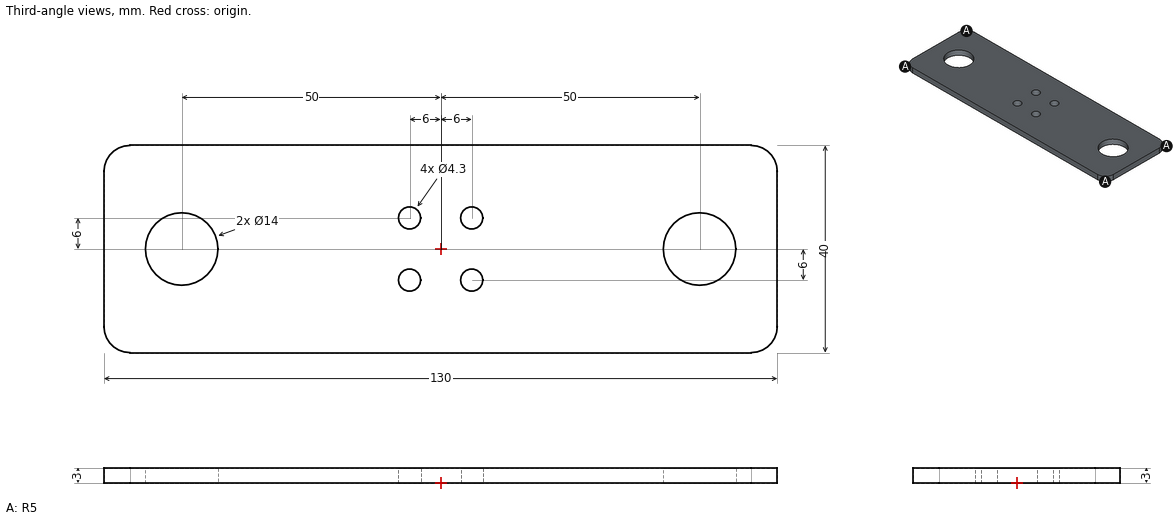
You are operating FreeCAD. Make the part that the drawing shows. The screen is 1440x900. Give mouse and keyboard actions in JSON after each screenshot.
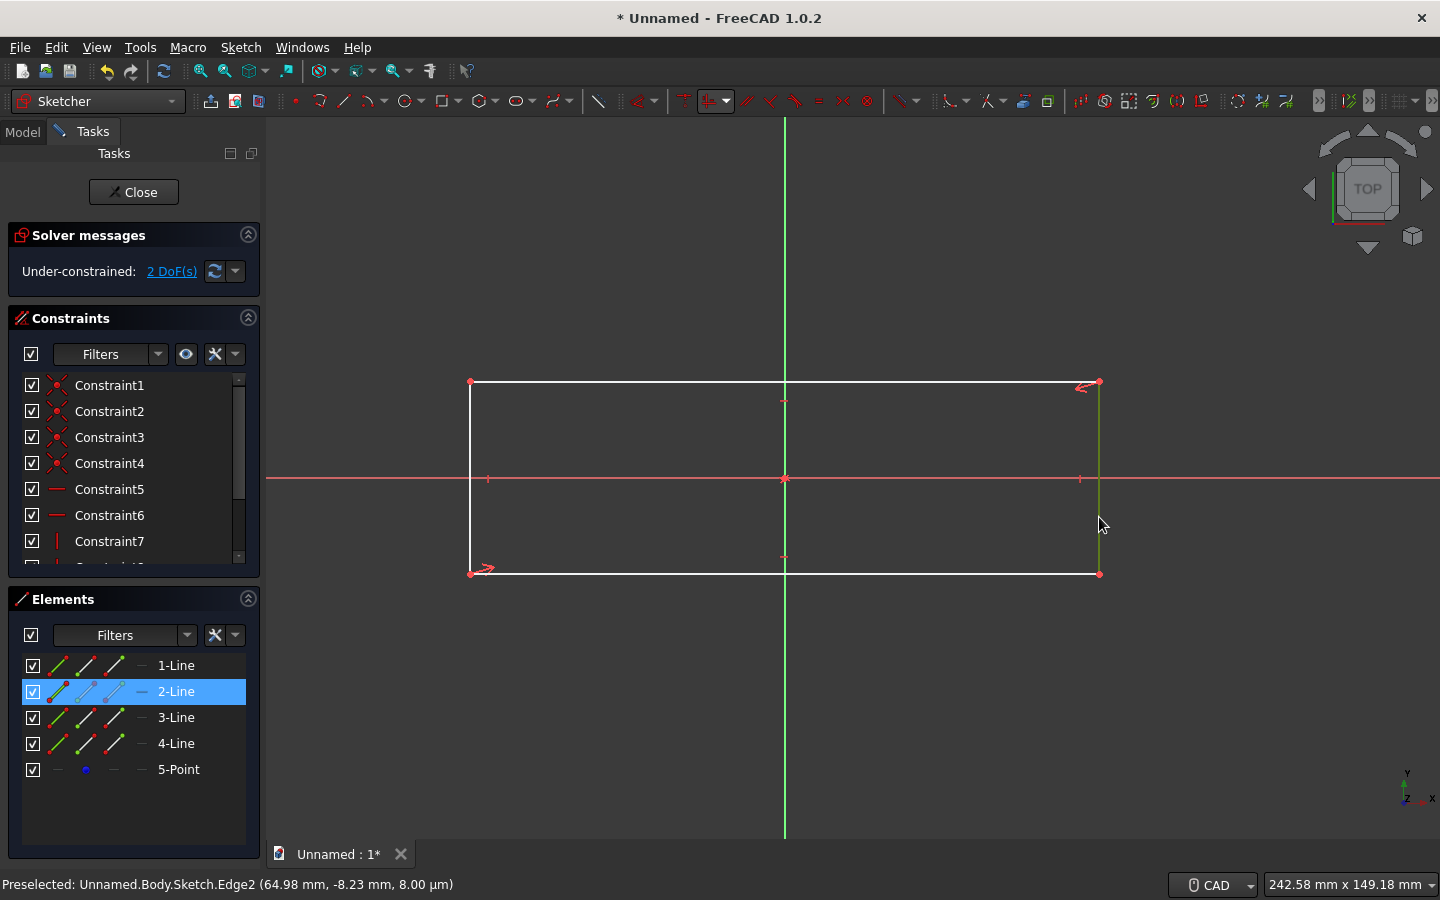
{"action": "key", "text": "i"}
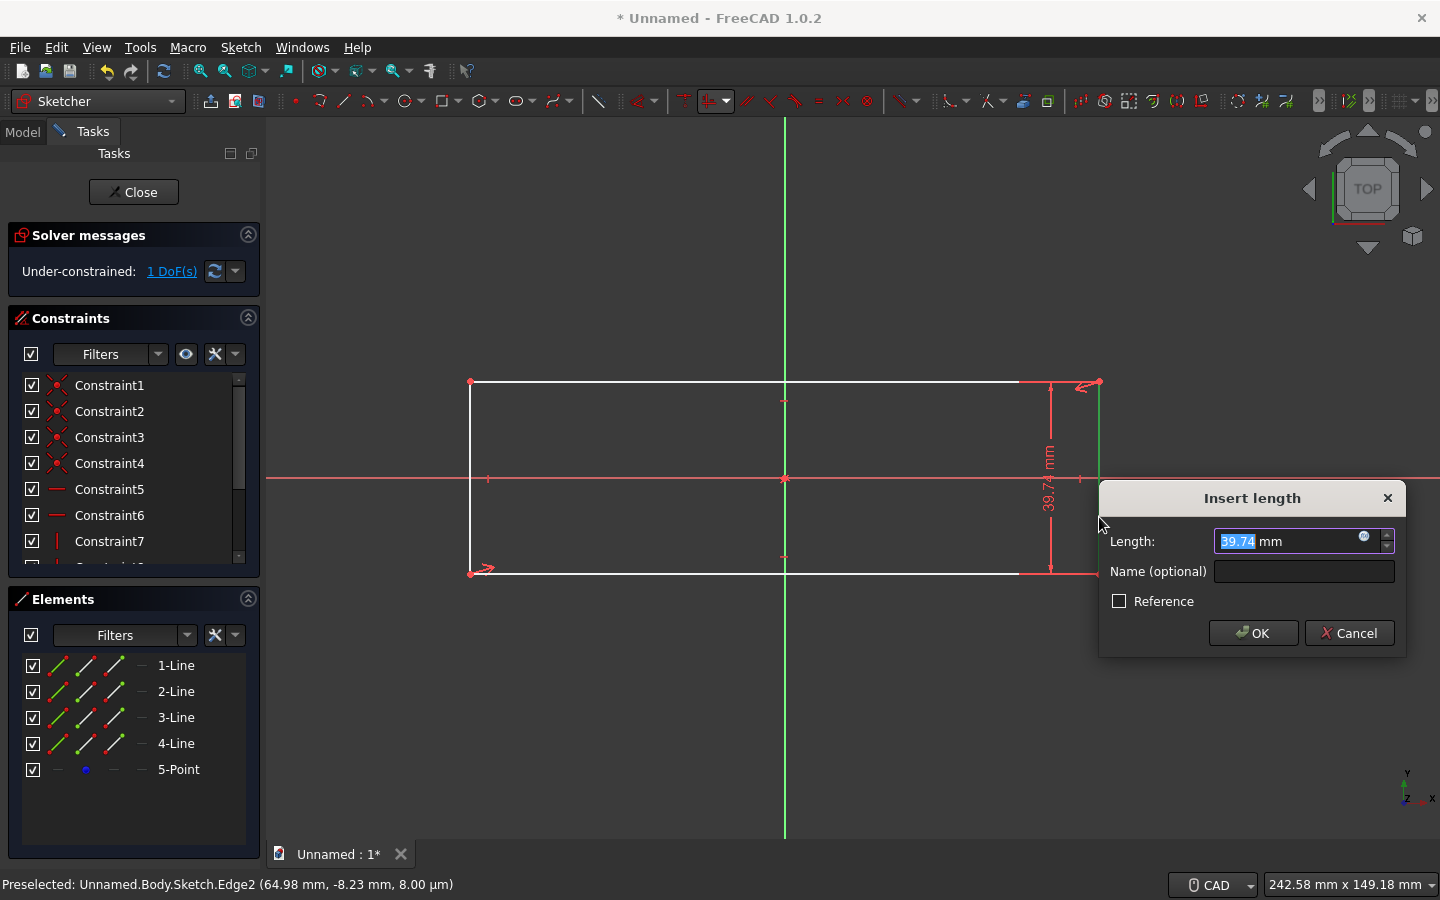
{"action": "type", "text": "40"}
{"action": "key", "text": "Return"}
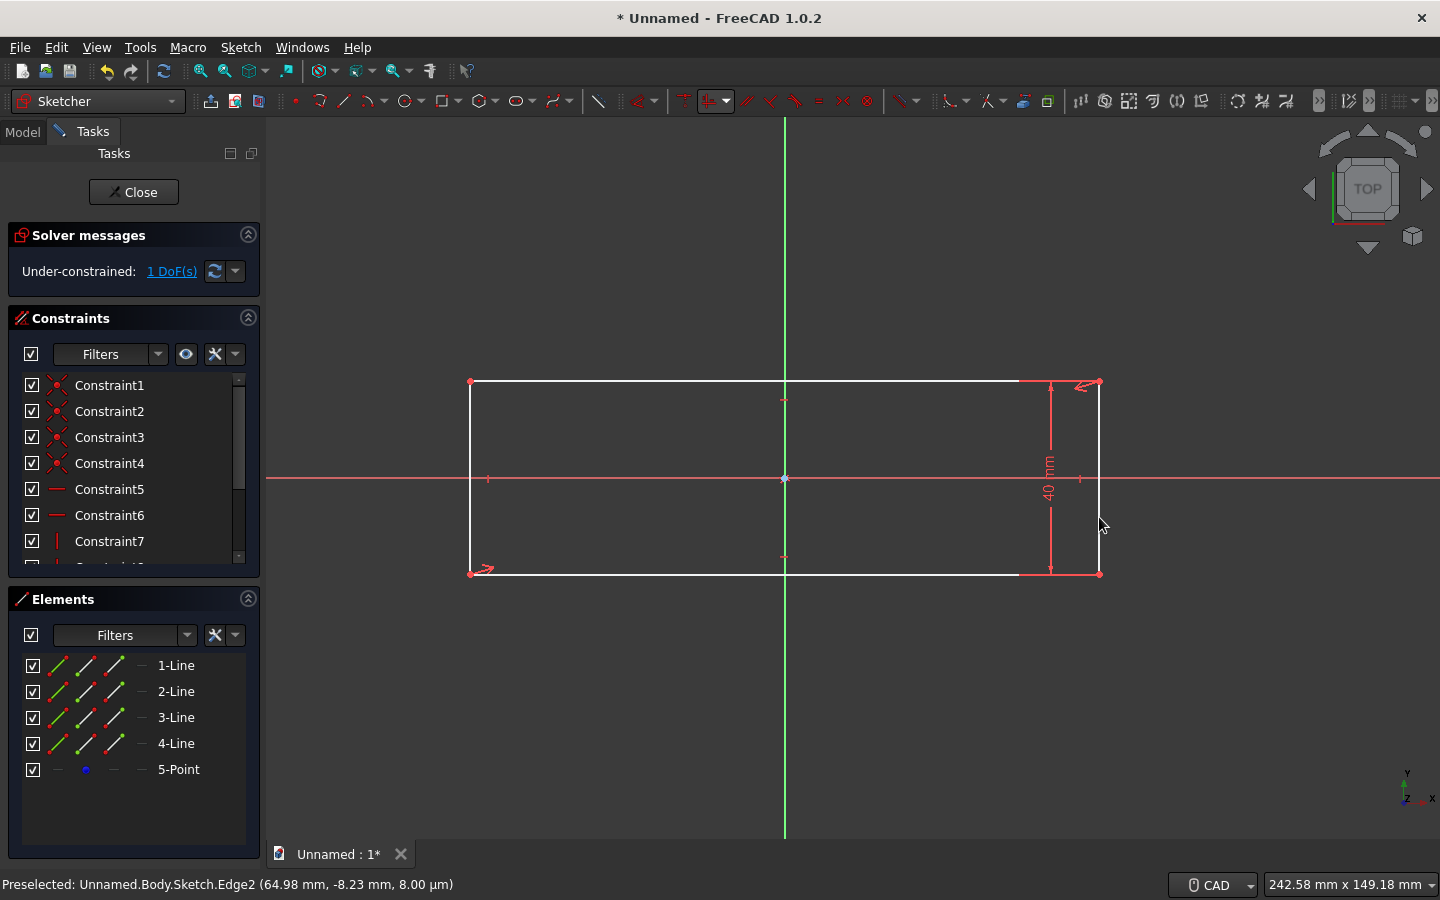
{"action": "left_click", "coordinate": [659, 575]}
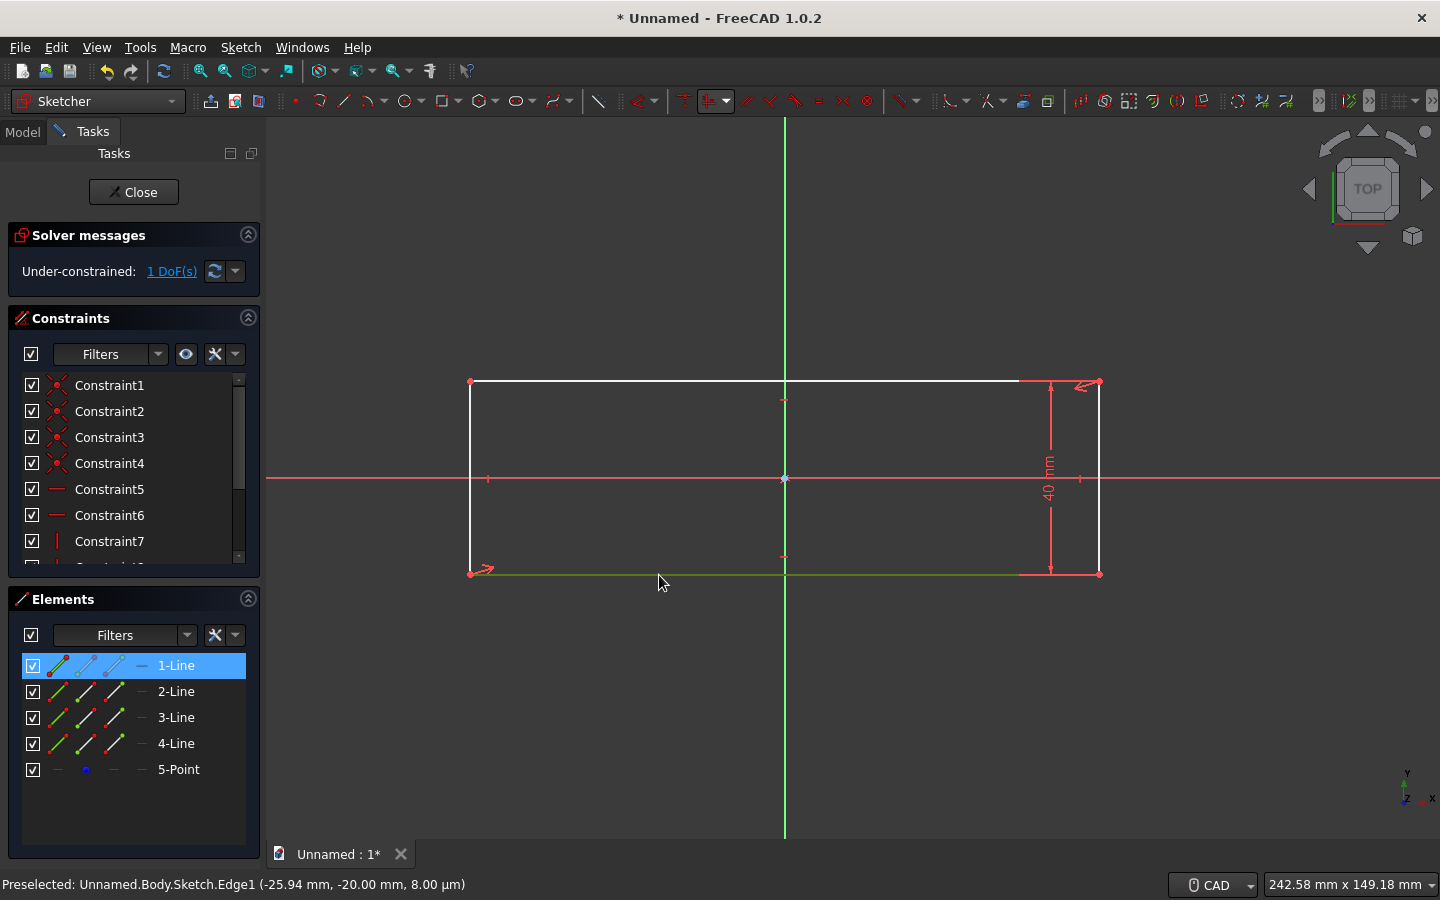
{"action": "key", "text": "l"}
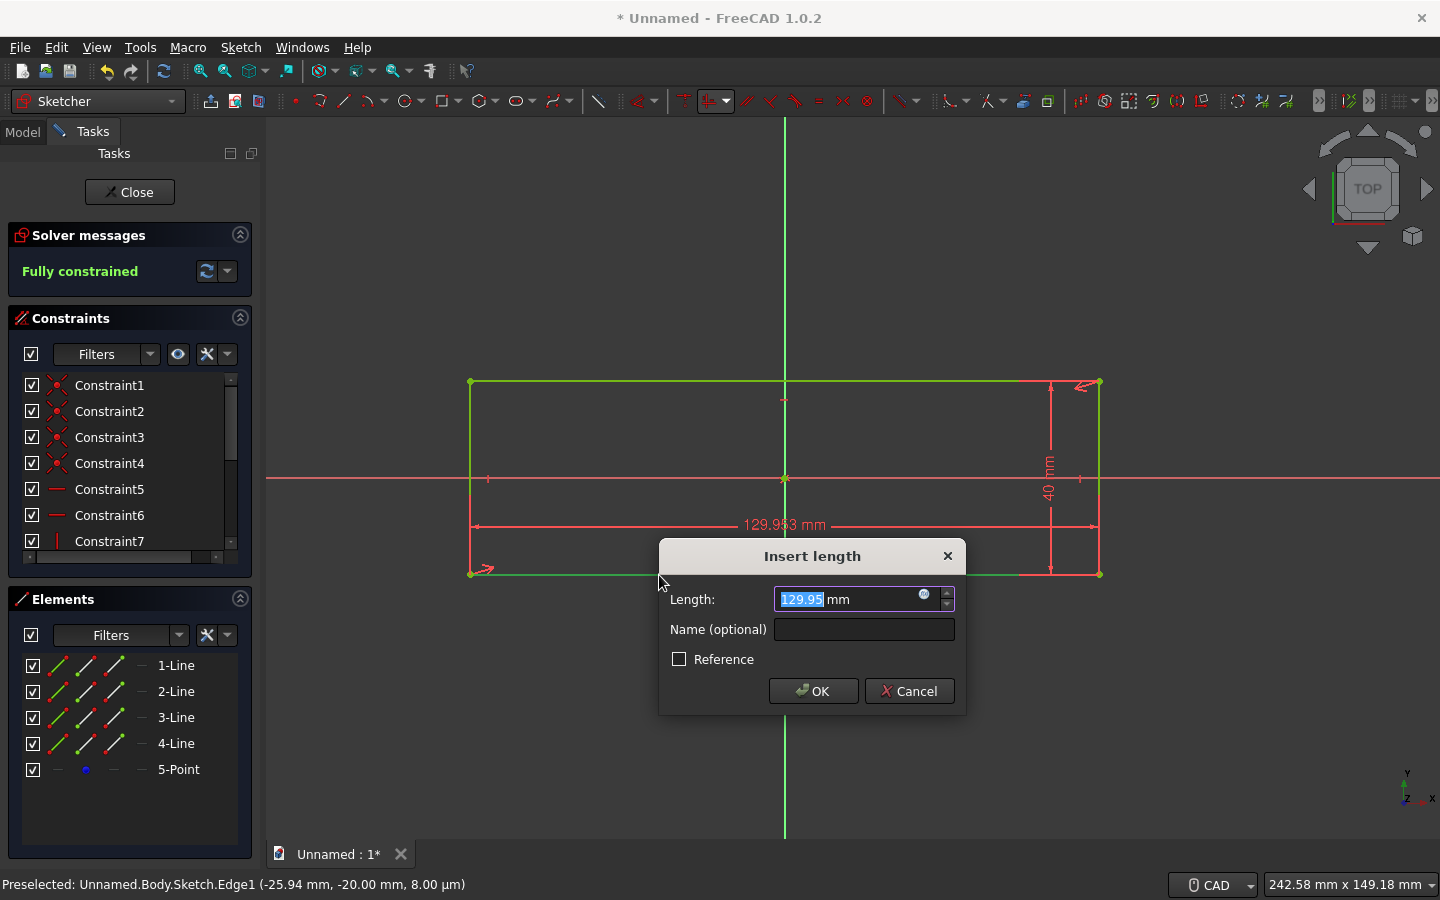
{"action": "type", "text": "130"}
{"action": "key", "text": "Return"}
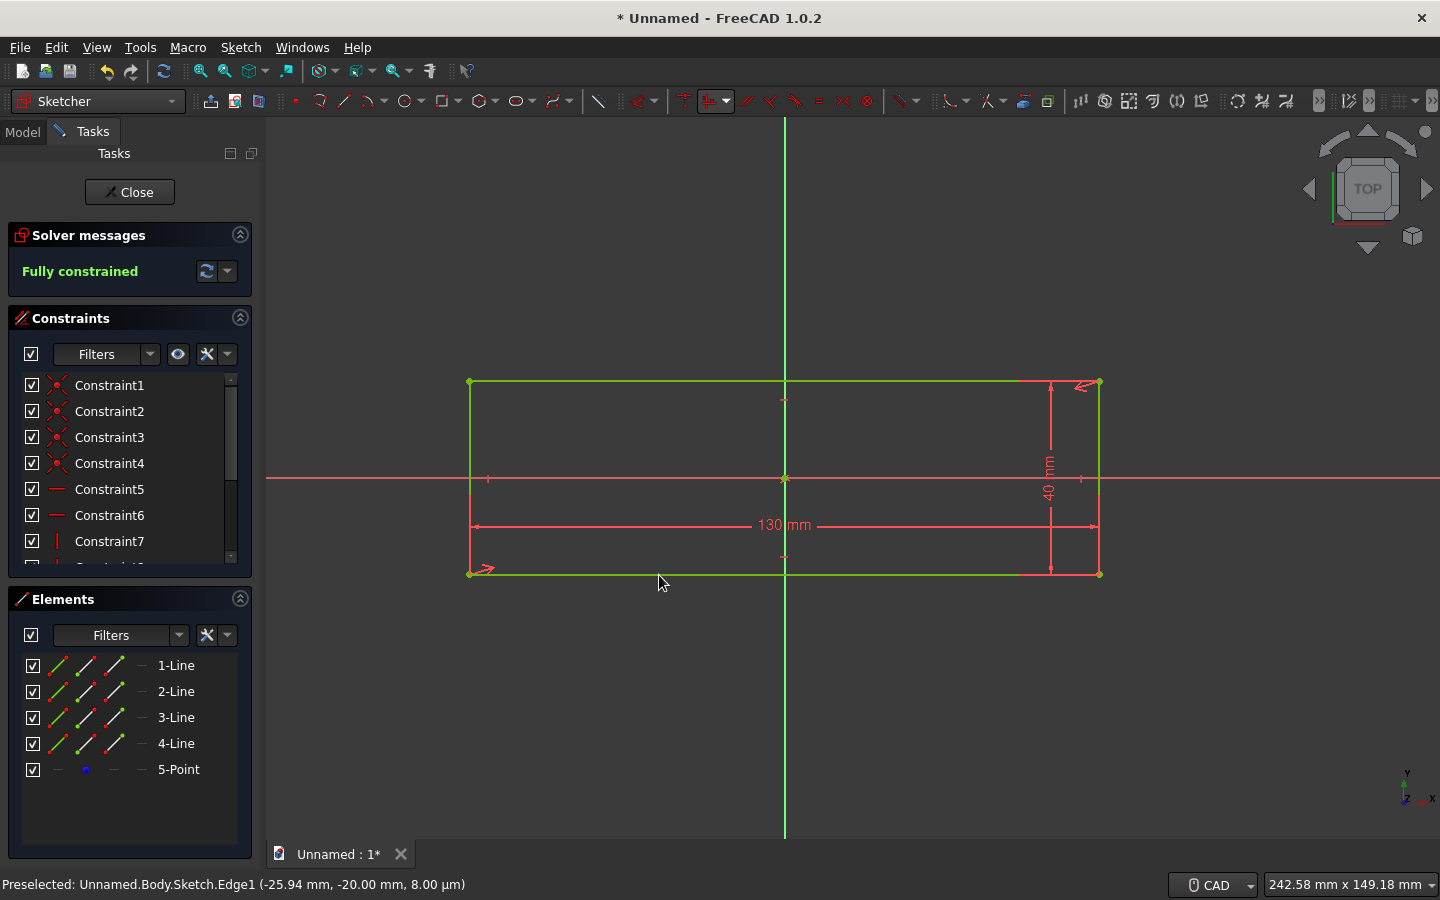
{"action": "left_click", "coordinate": [130, 192]}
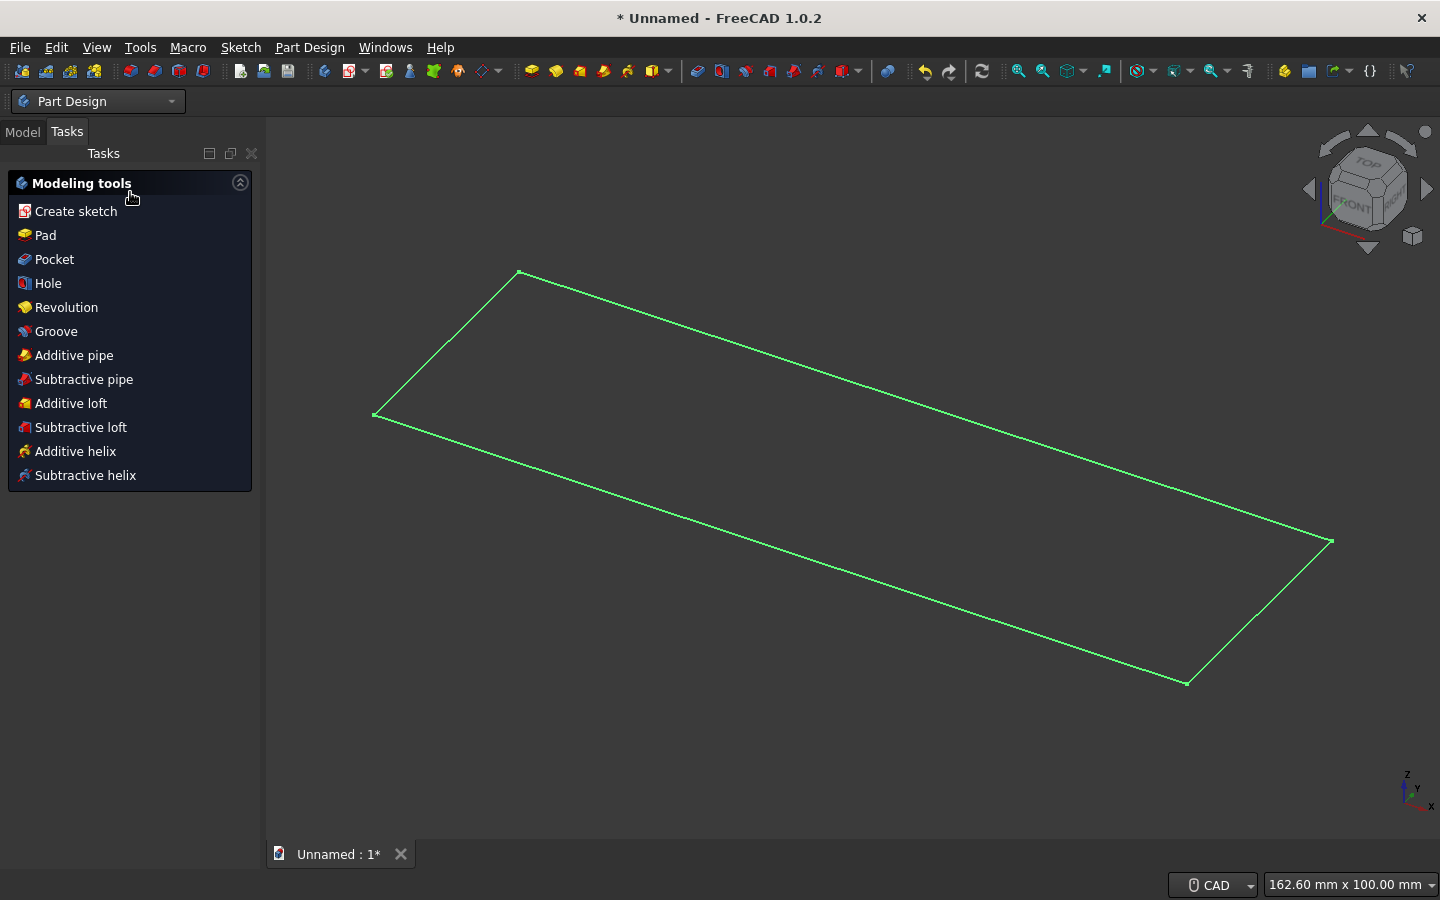
{"action": "left_click", "coordinate": [532, 72]}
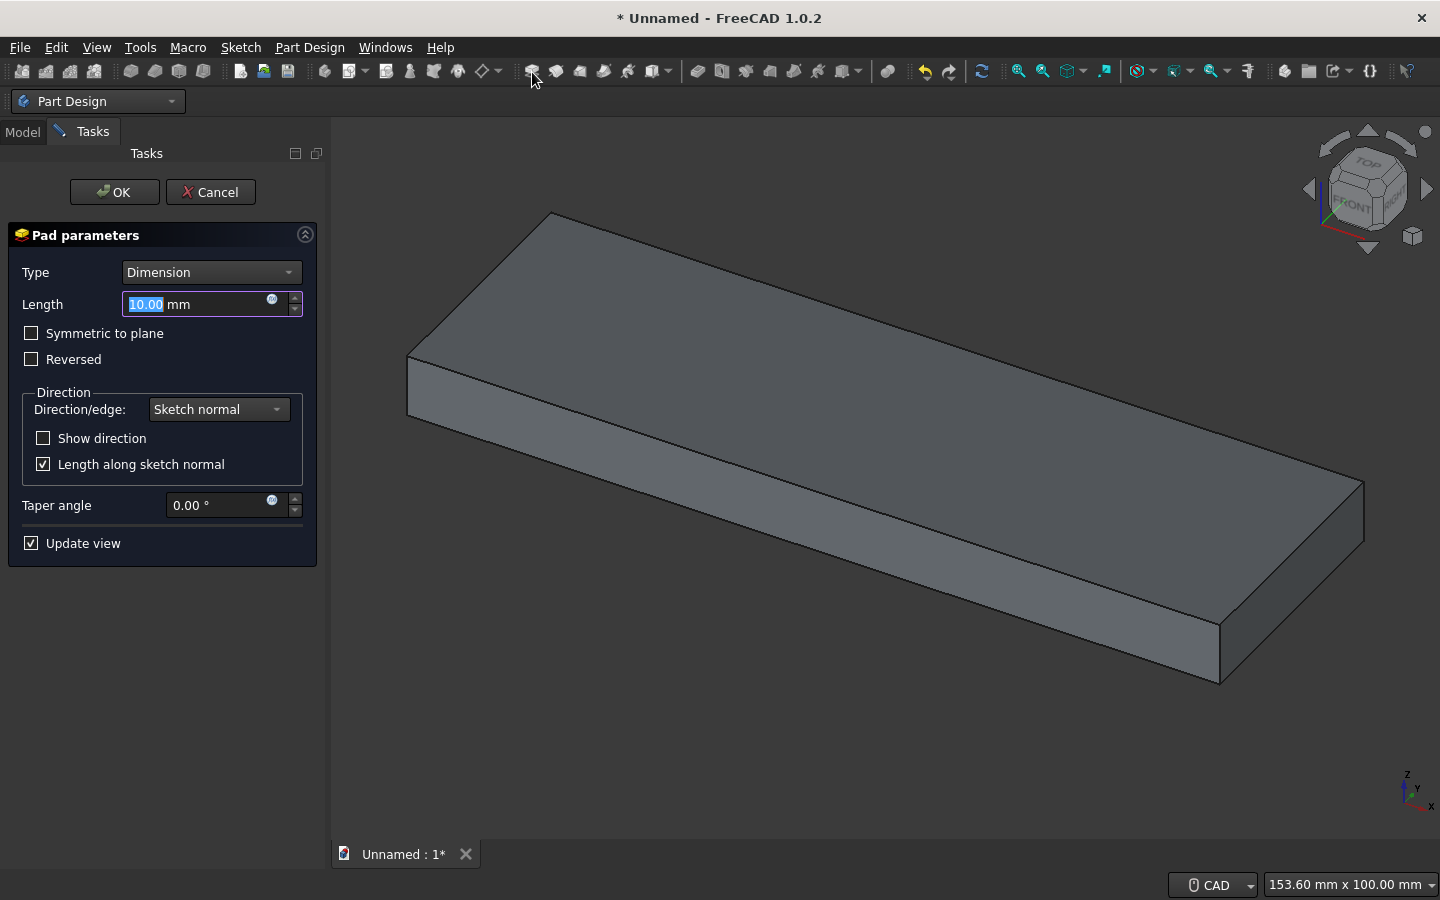
{"action": "type", "text": "3"}
{"action": "key", "text": "Tab"}